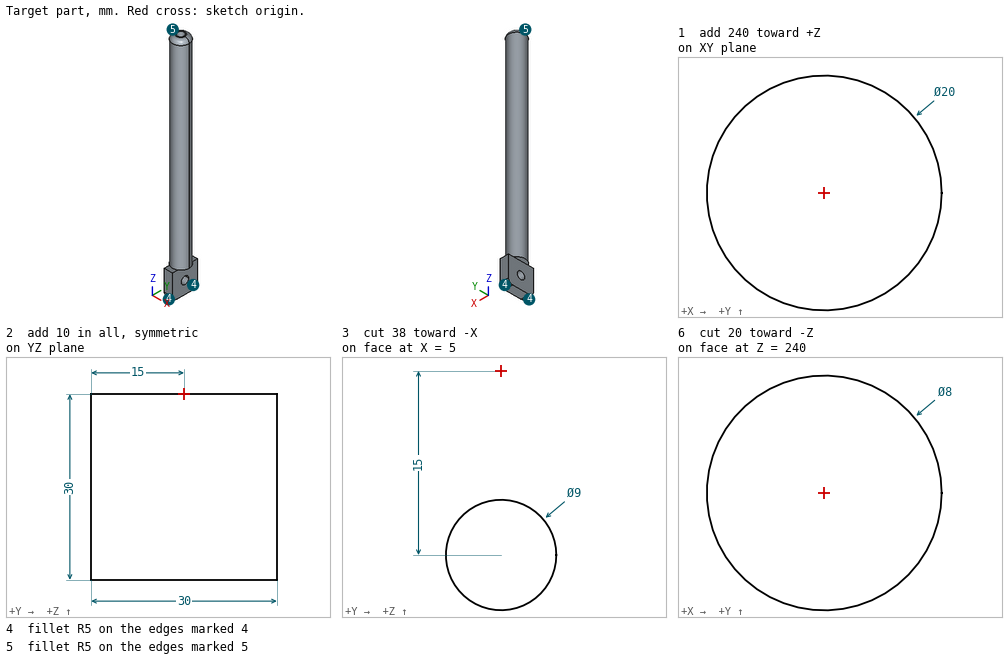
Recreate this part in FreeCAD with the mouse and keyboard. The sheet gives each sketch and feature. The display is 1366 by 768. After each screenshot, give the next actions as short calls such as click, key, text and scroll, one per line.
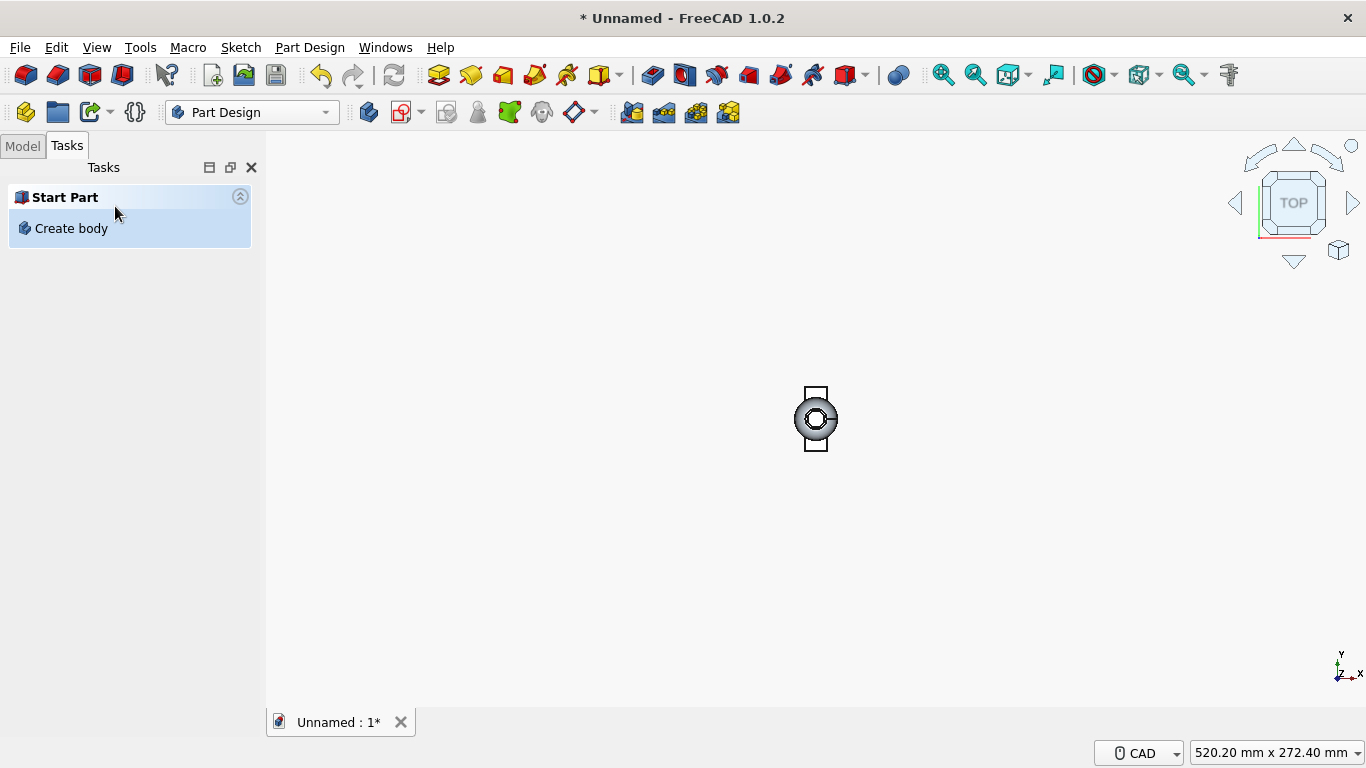
key(0)